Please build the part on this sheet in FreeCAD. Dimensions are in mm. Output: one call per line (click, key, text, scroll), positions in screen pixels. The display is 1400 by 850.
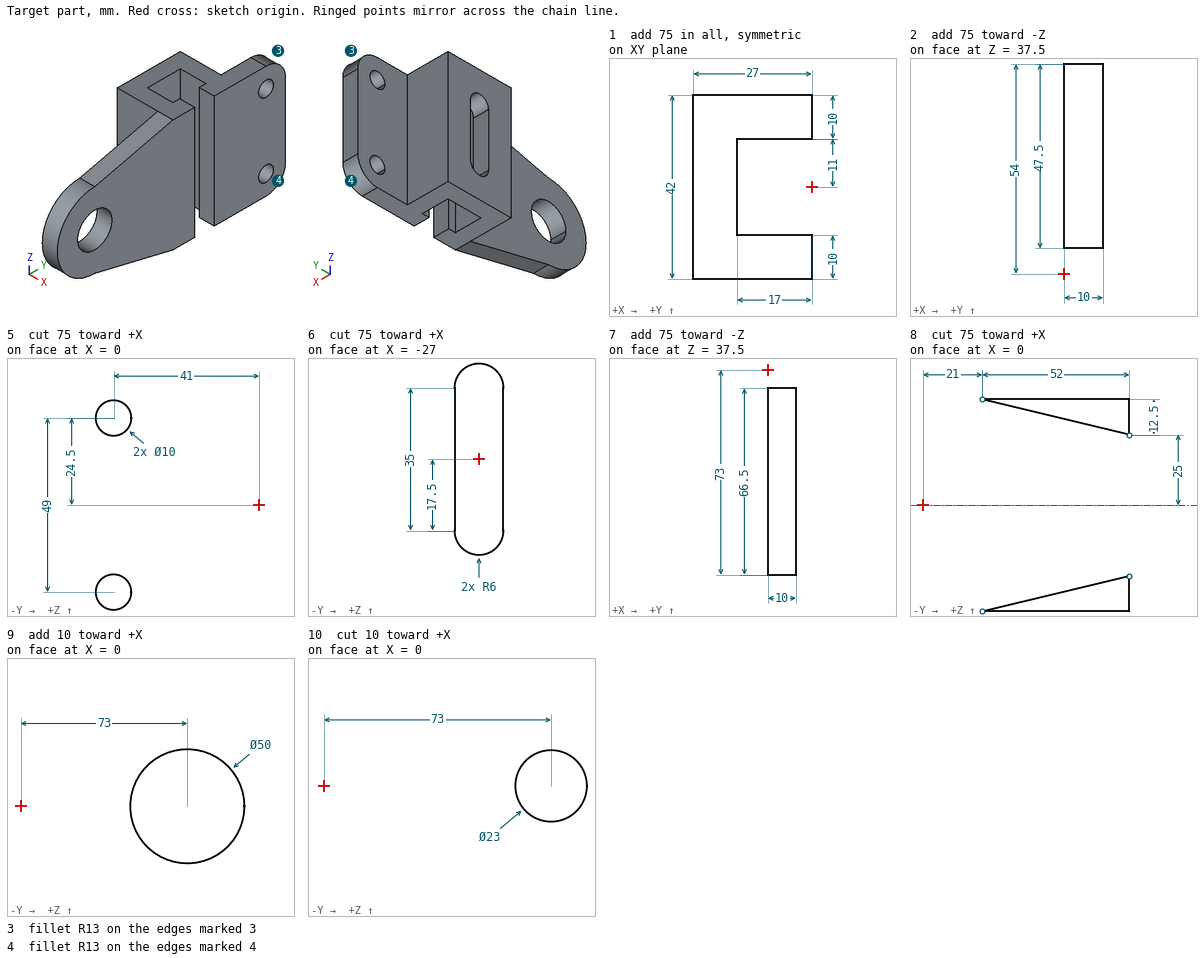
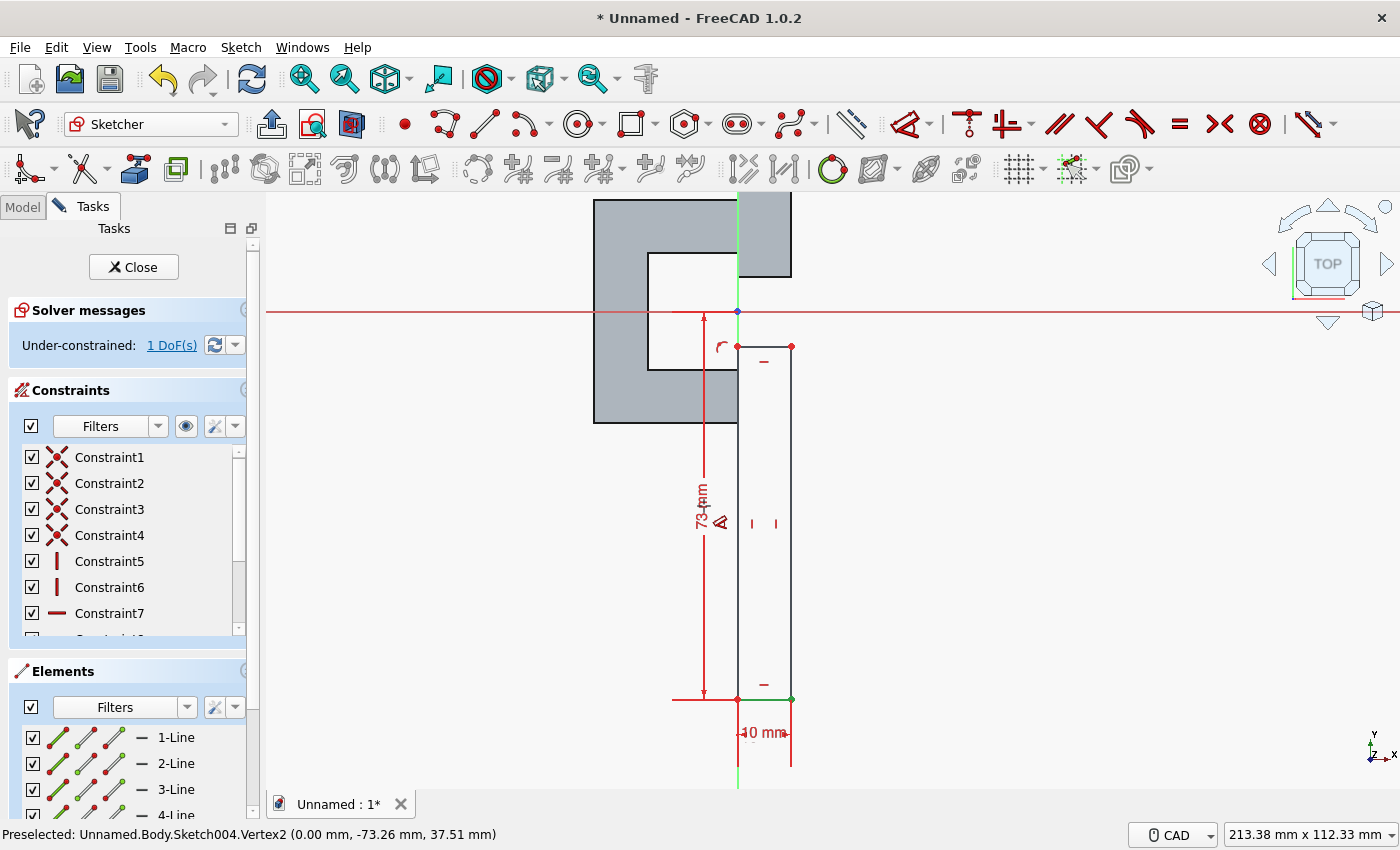
click(738, 453)
click(704, 442)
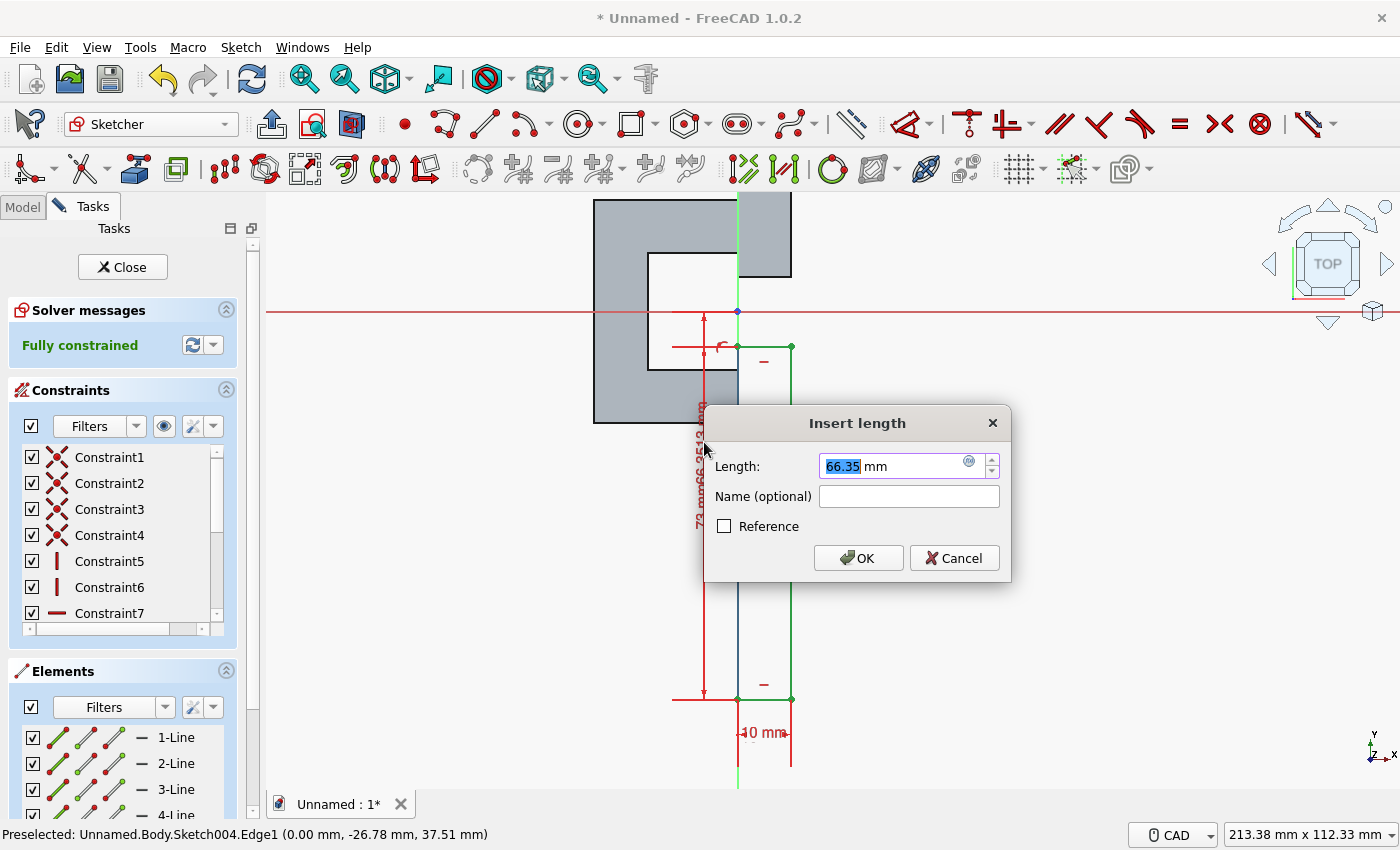
text(66.5)
key(Return)
key(Escape)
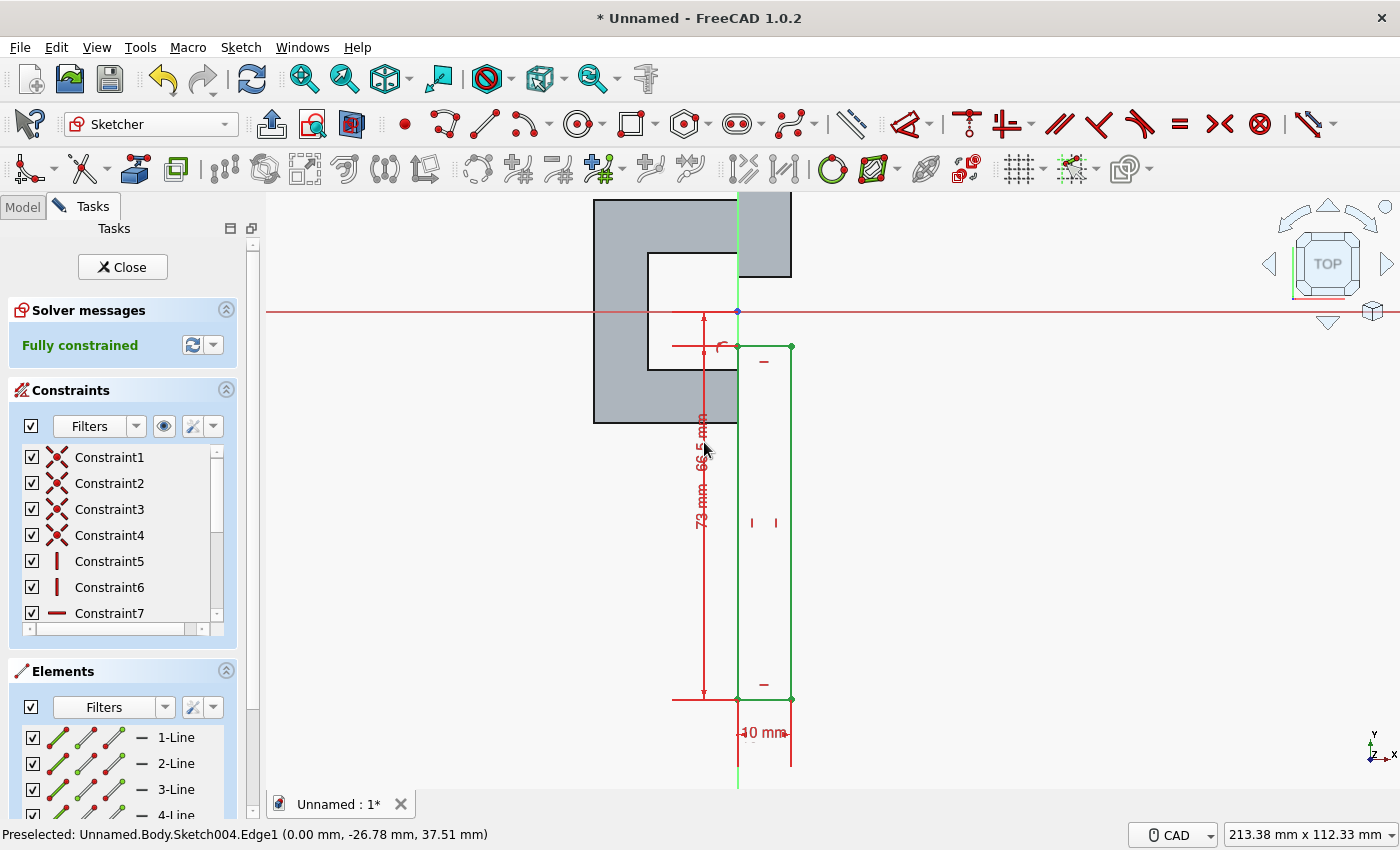
click(123, 267)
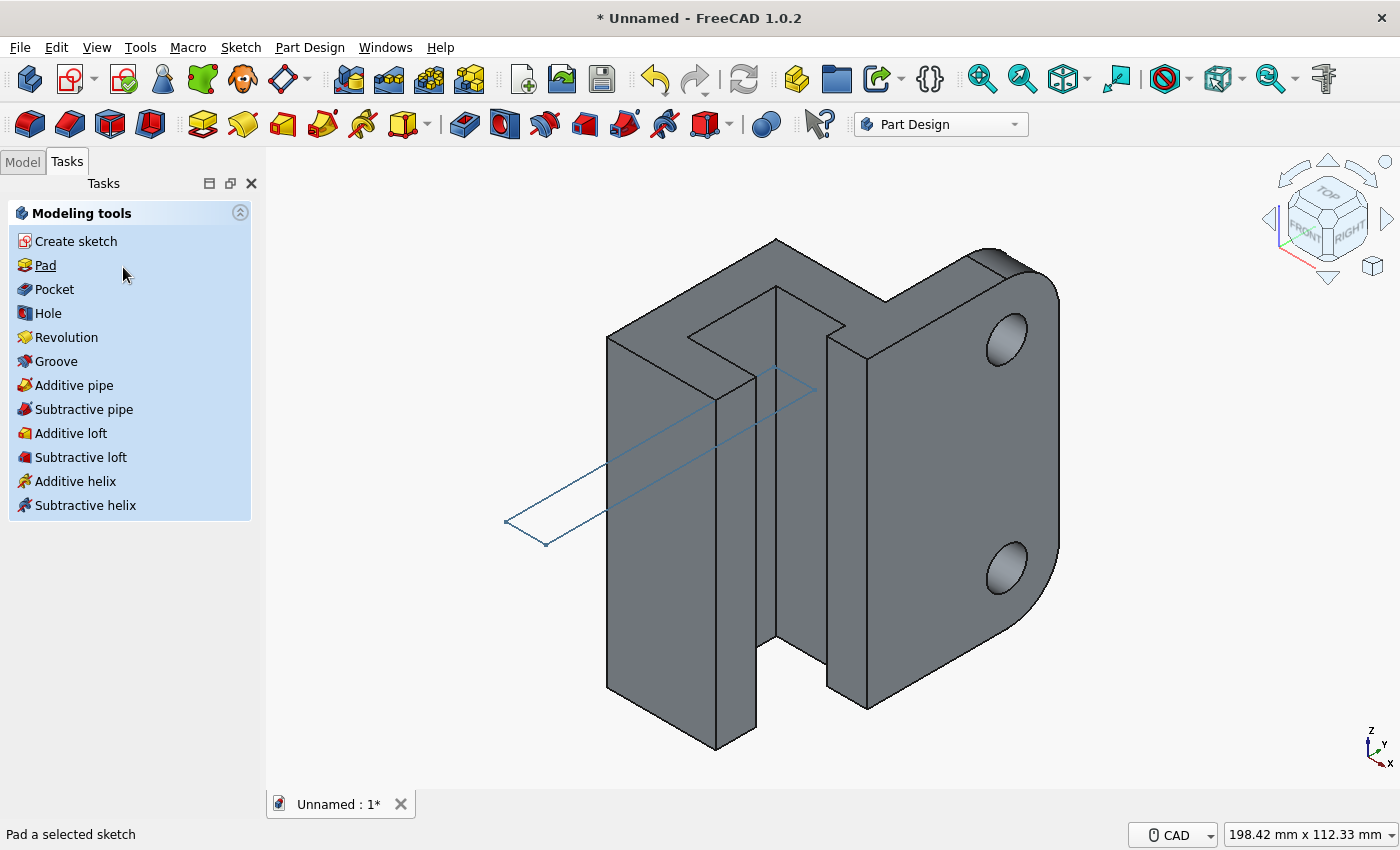
click(204, 124)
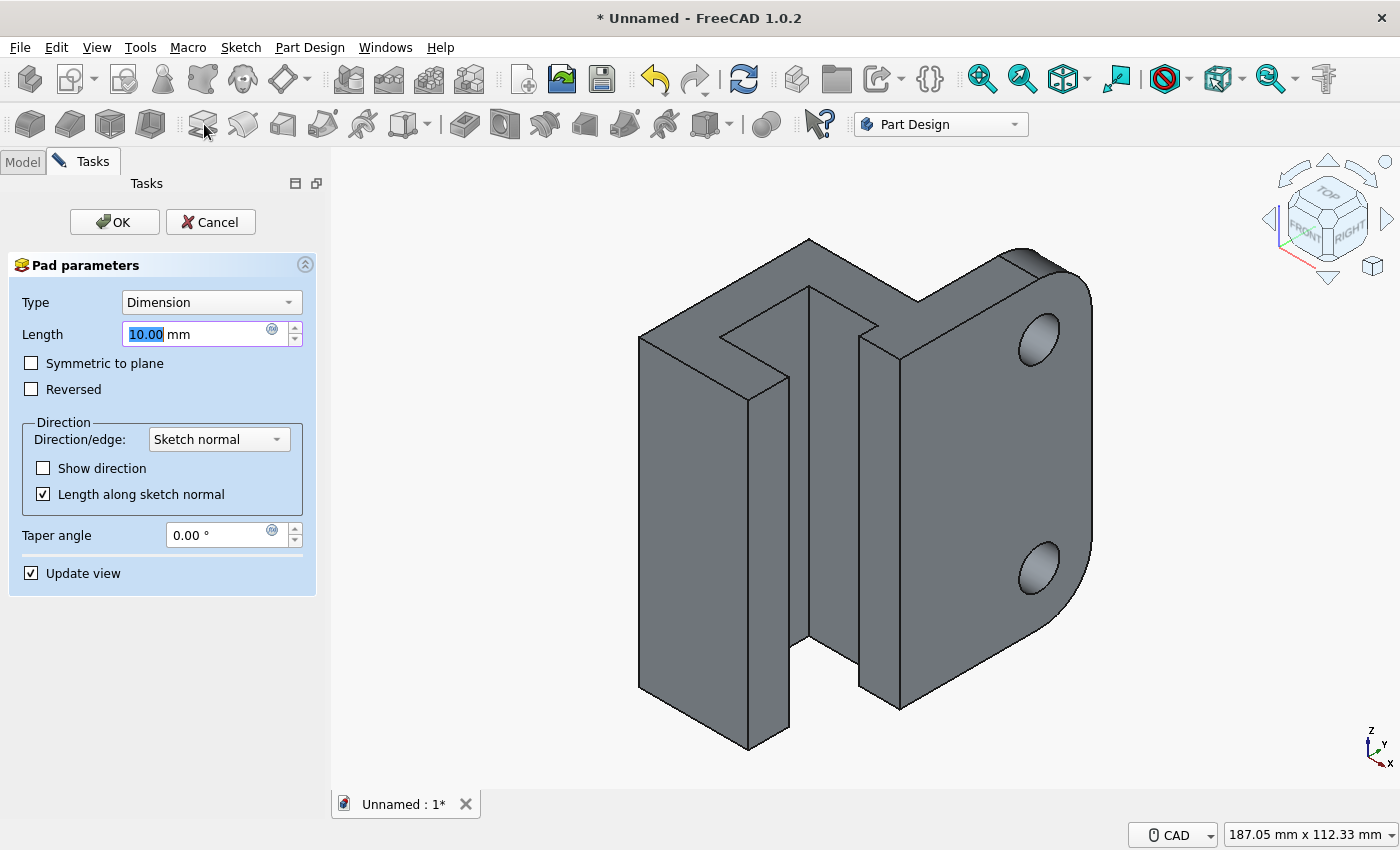
text(75)
key(Tab)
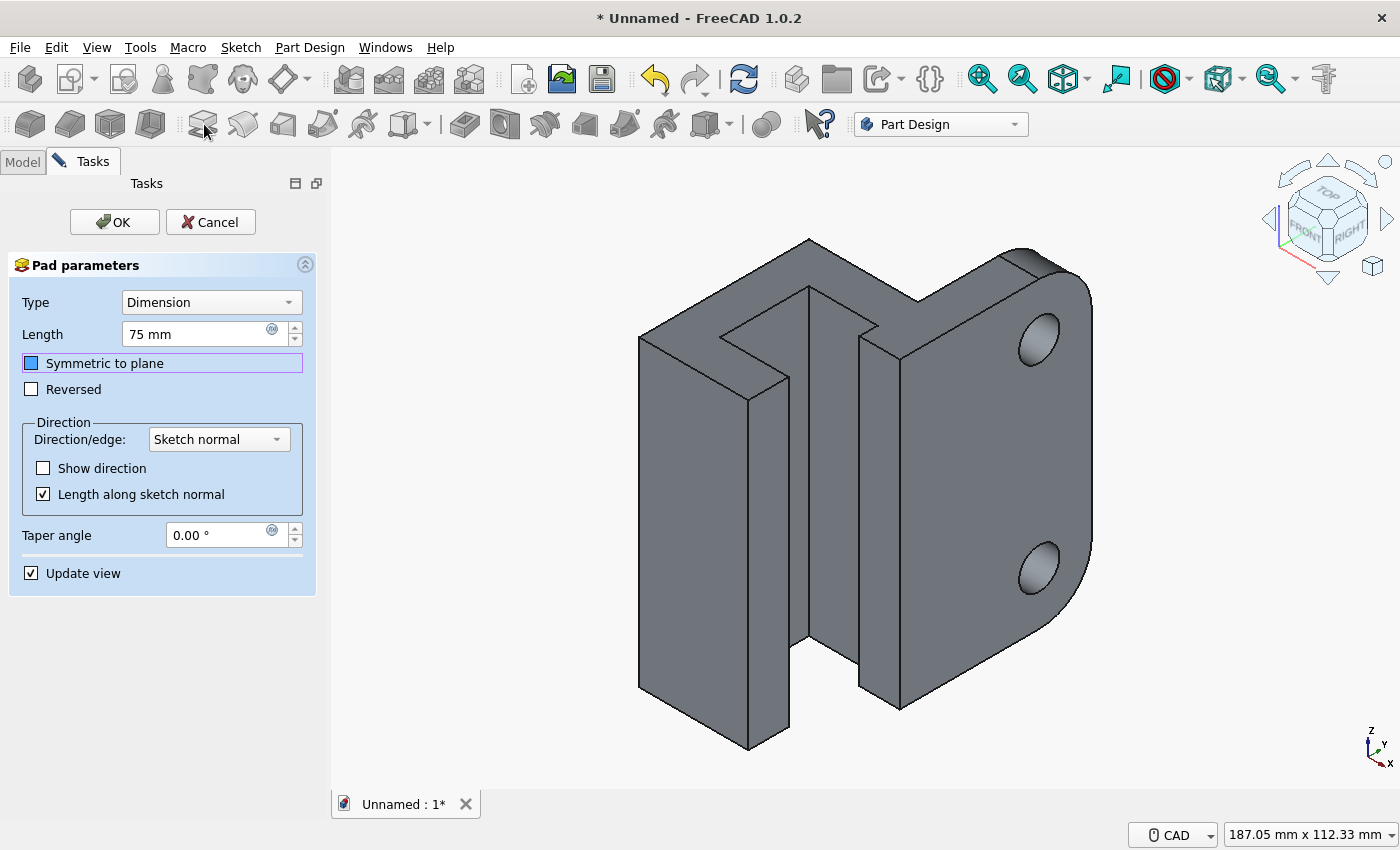
click(30, 389)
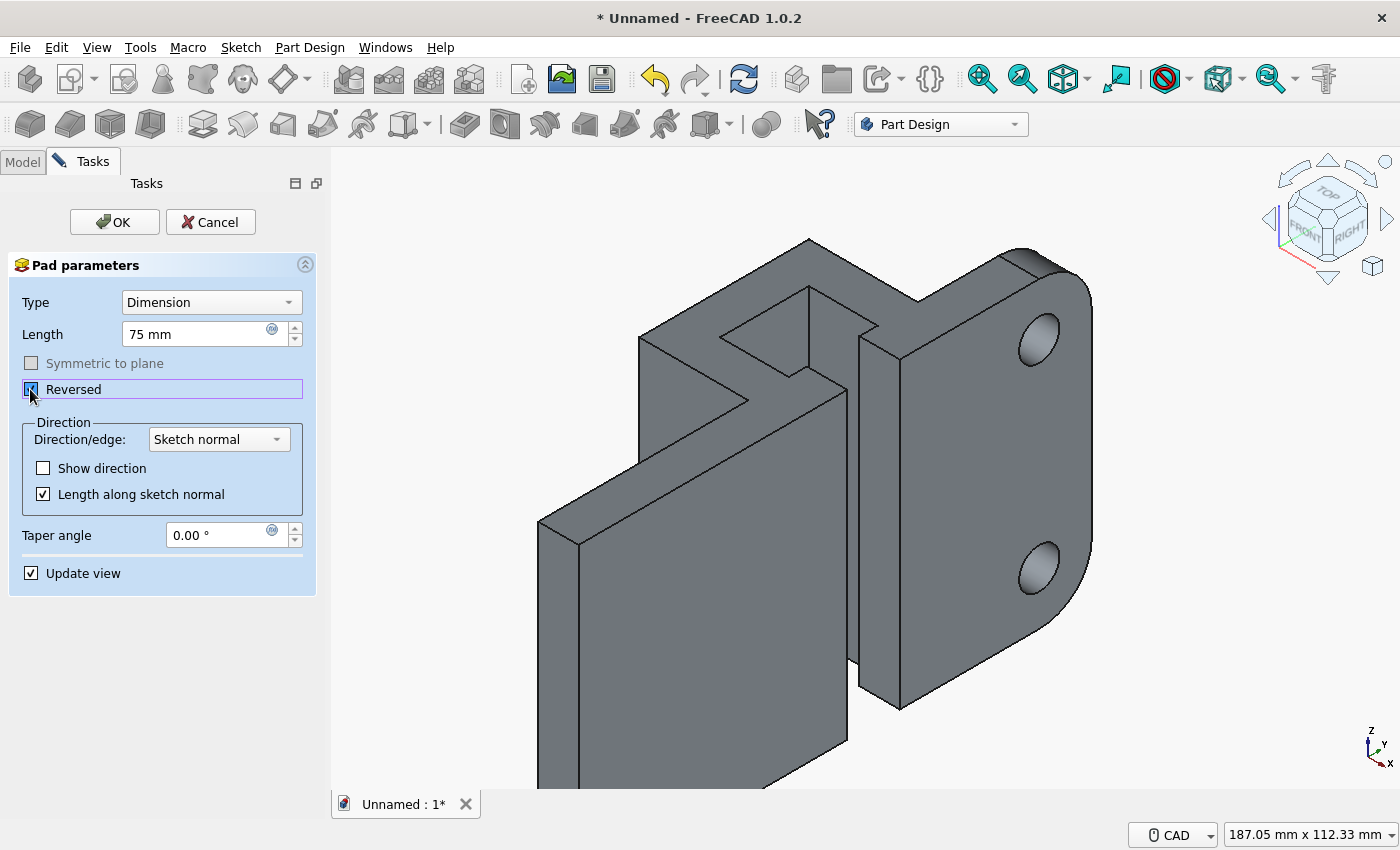
click(115, 222)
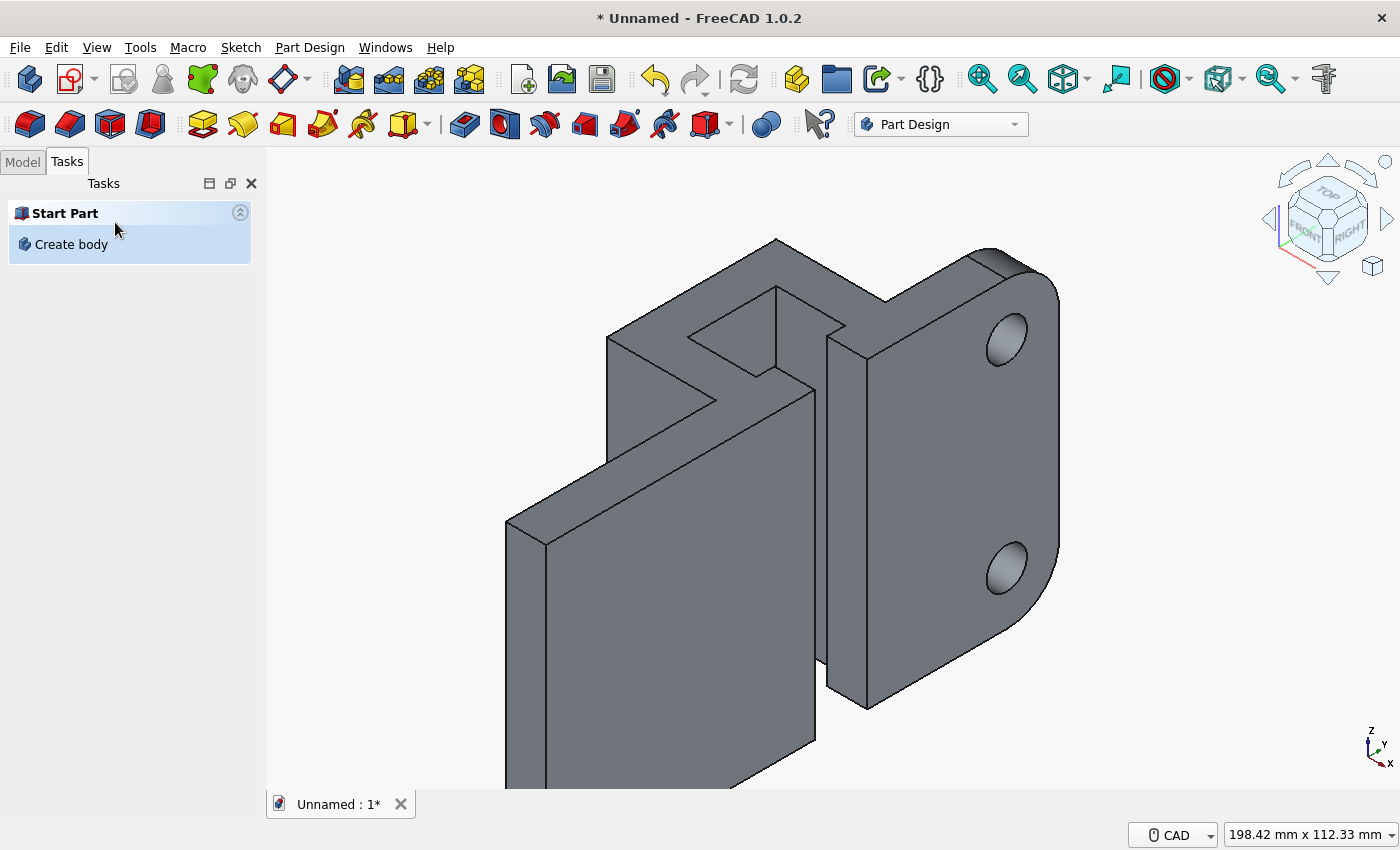
key(v)
key(f)